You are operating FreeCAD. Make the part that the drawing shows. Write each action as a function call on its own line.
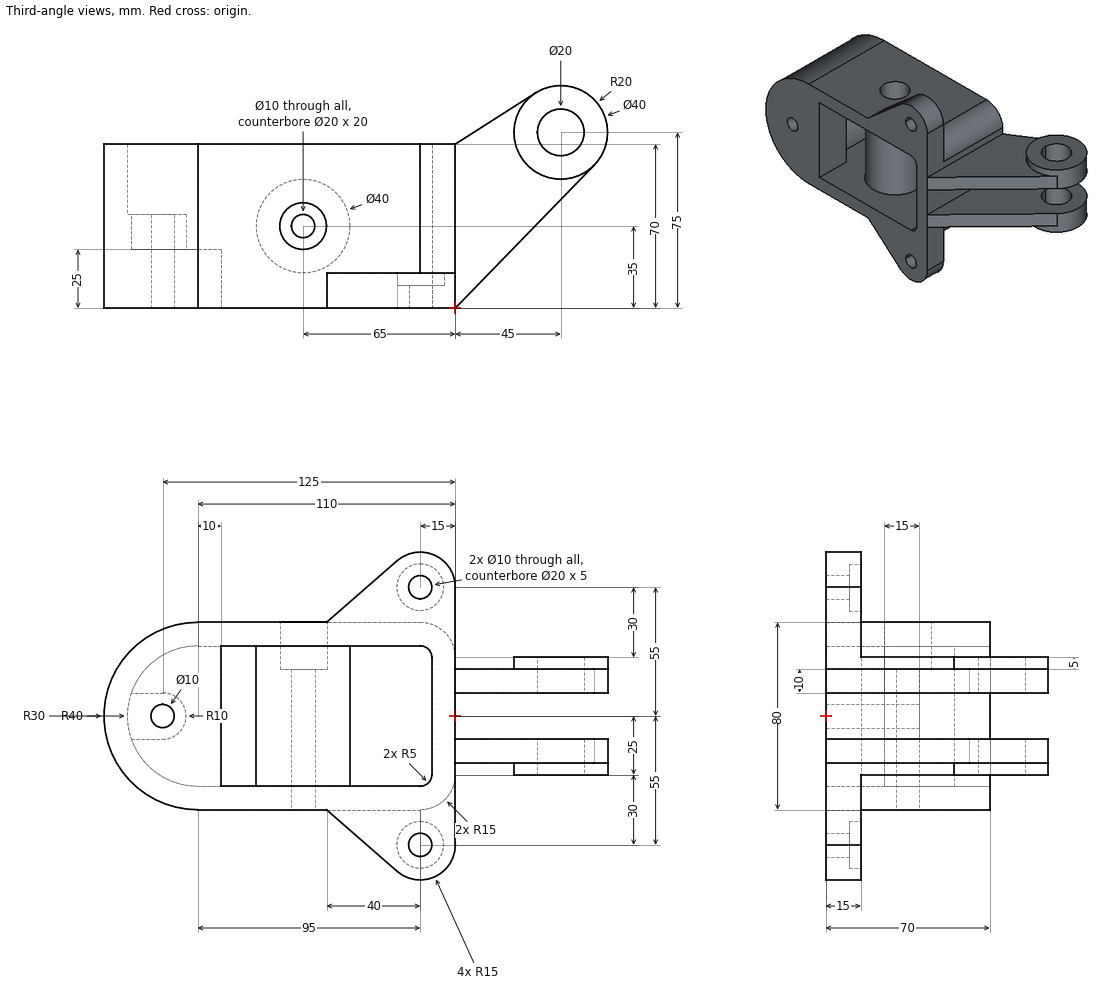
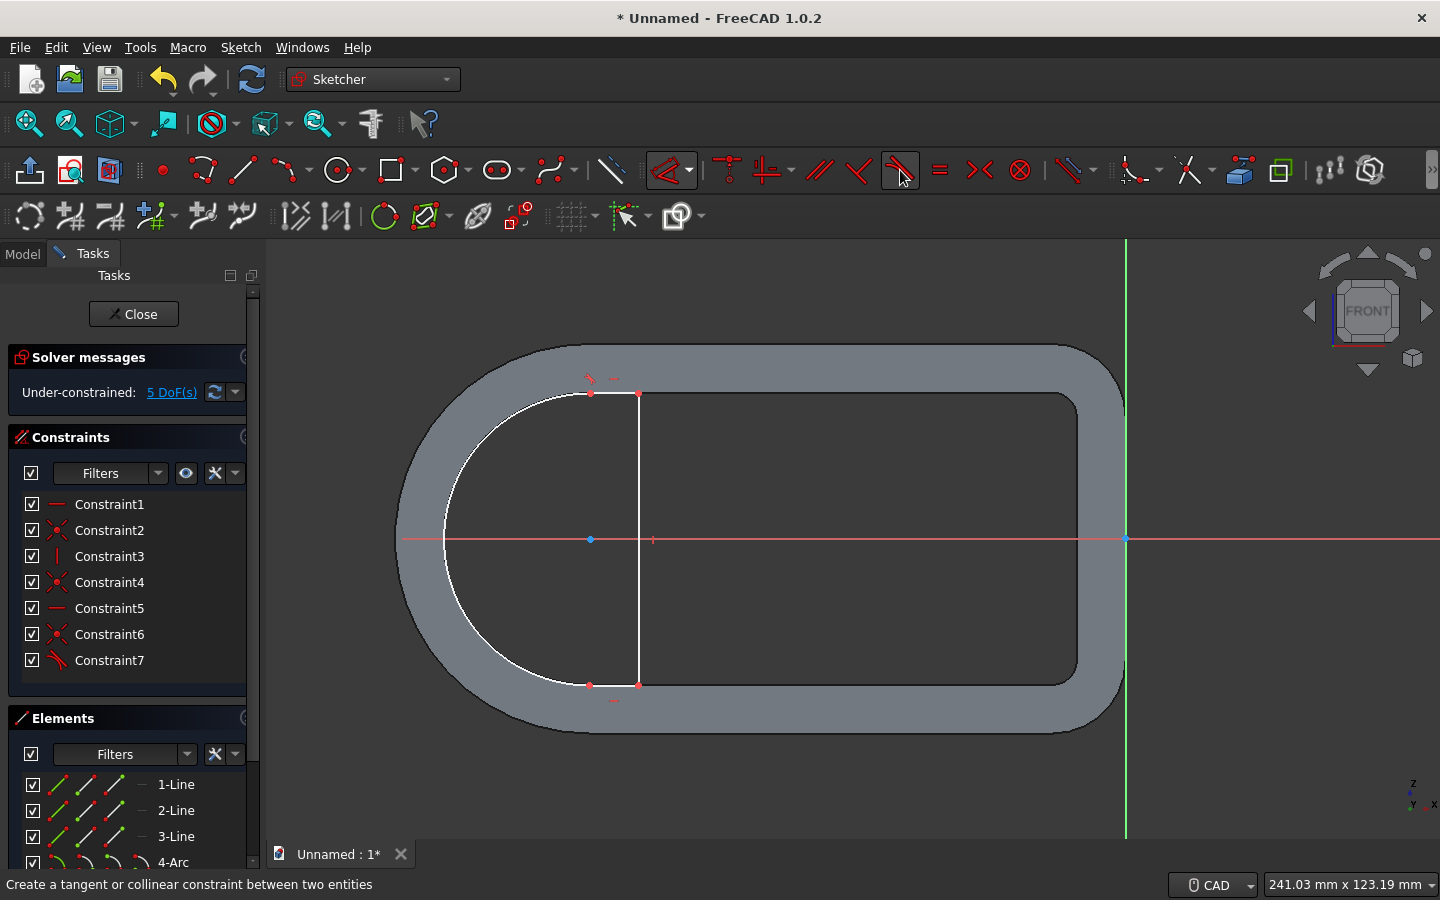
click(624, 686)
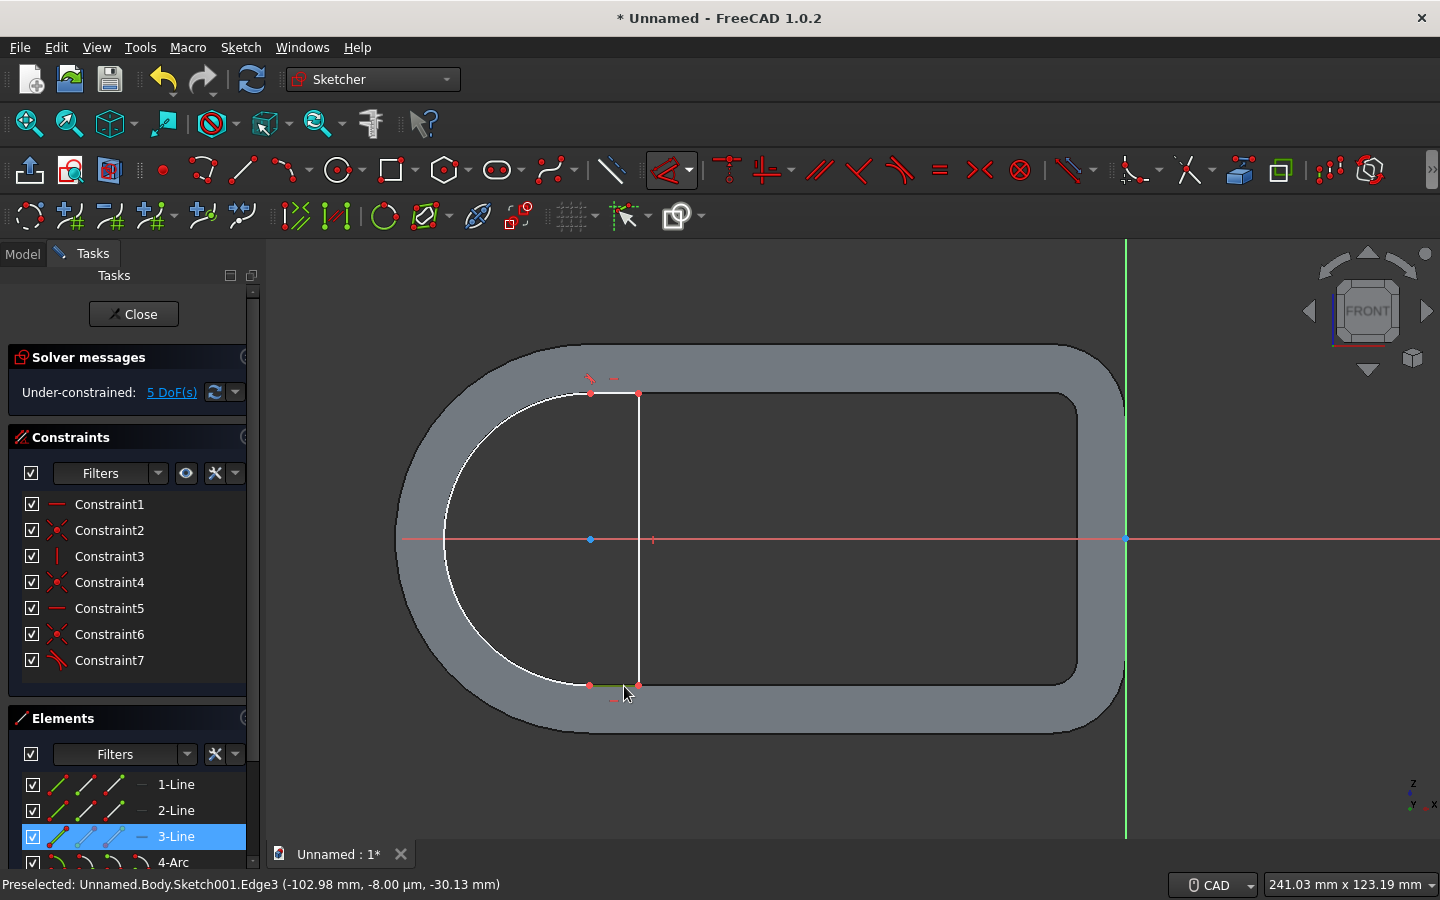
click(472, 454)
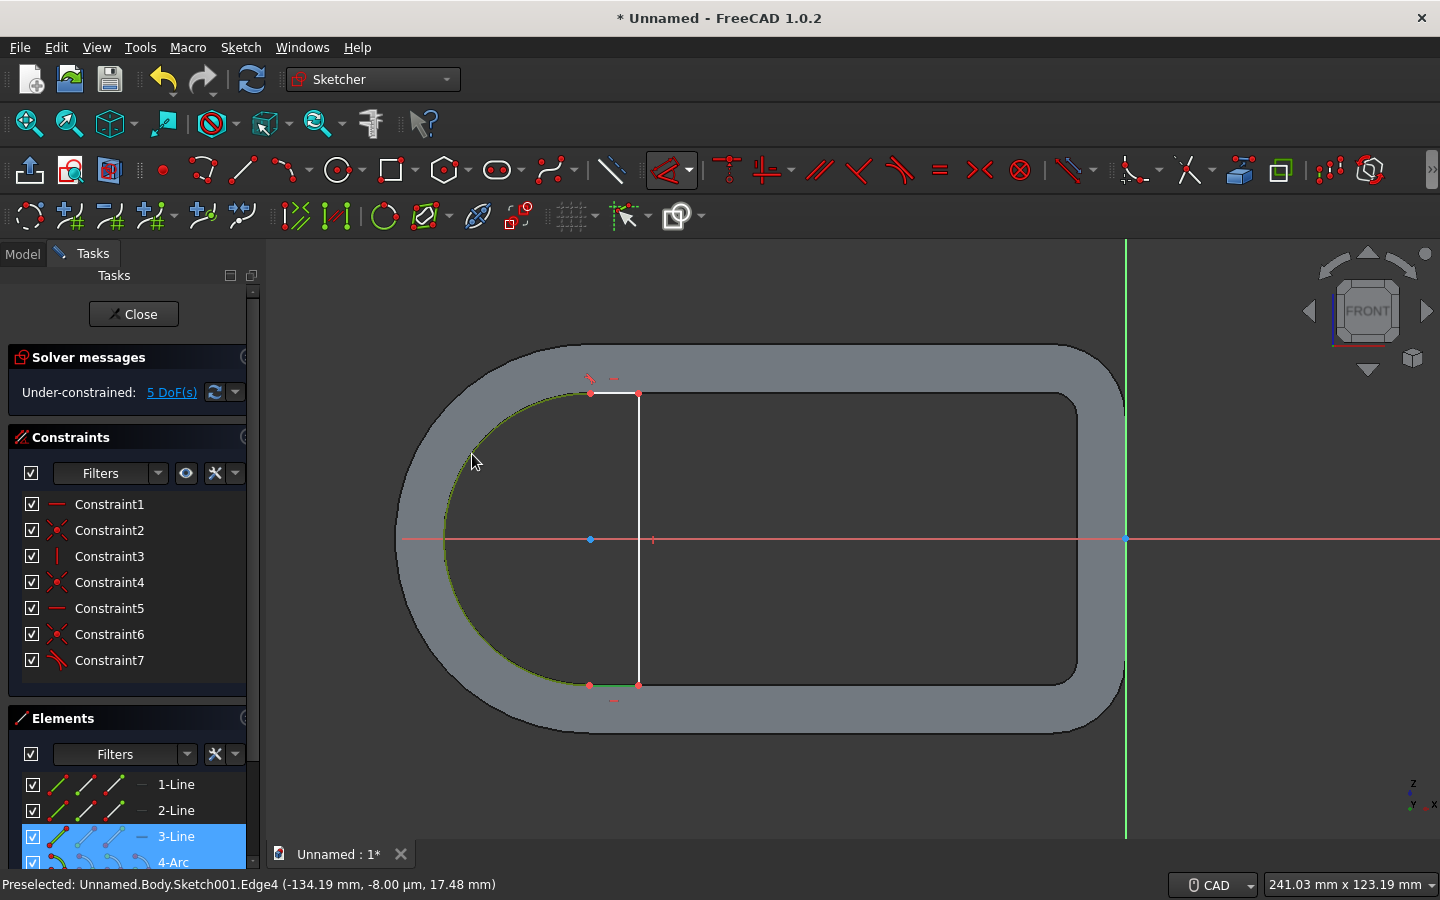
key(t)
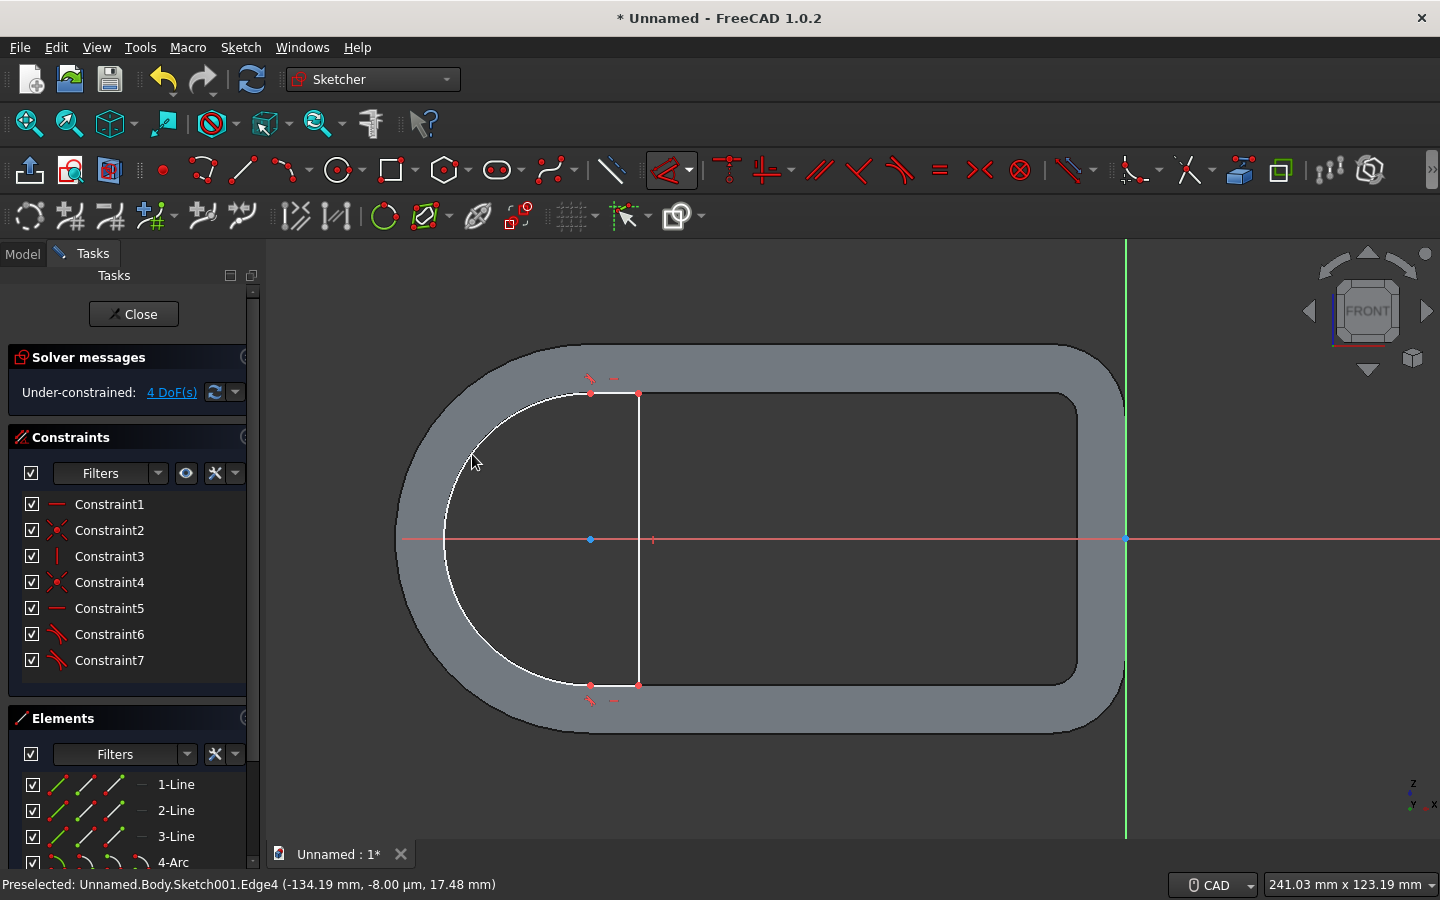
click(590, 539)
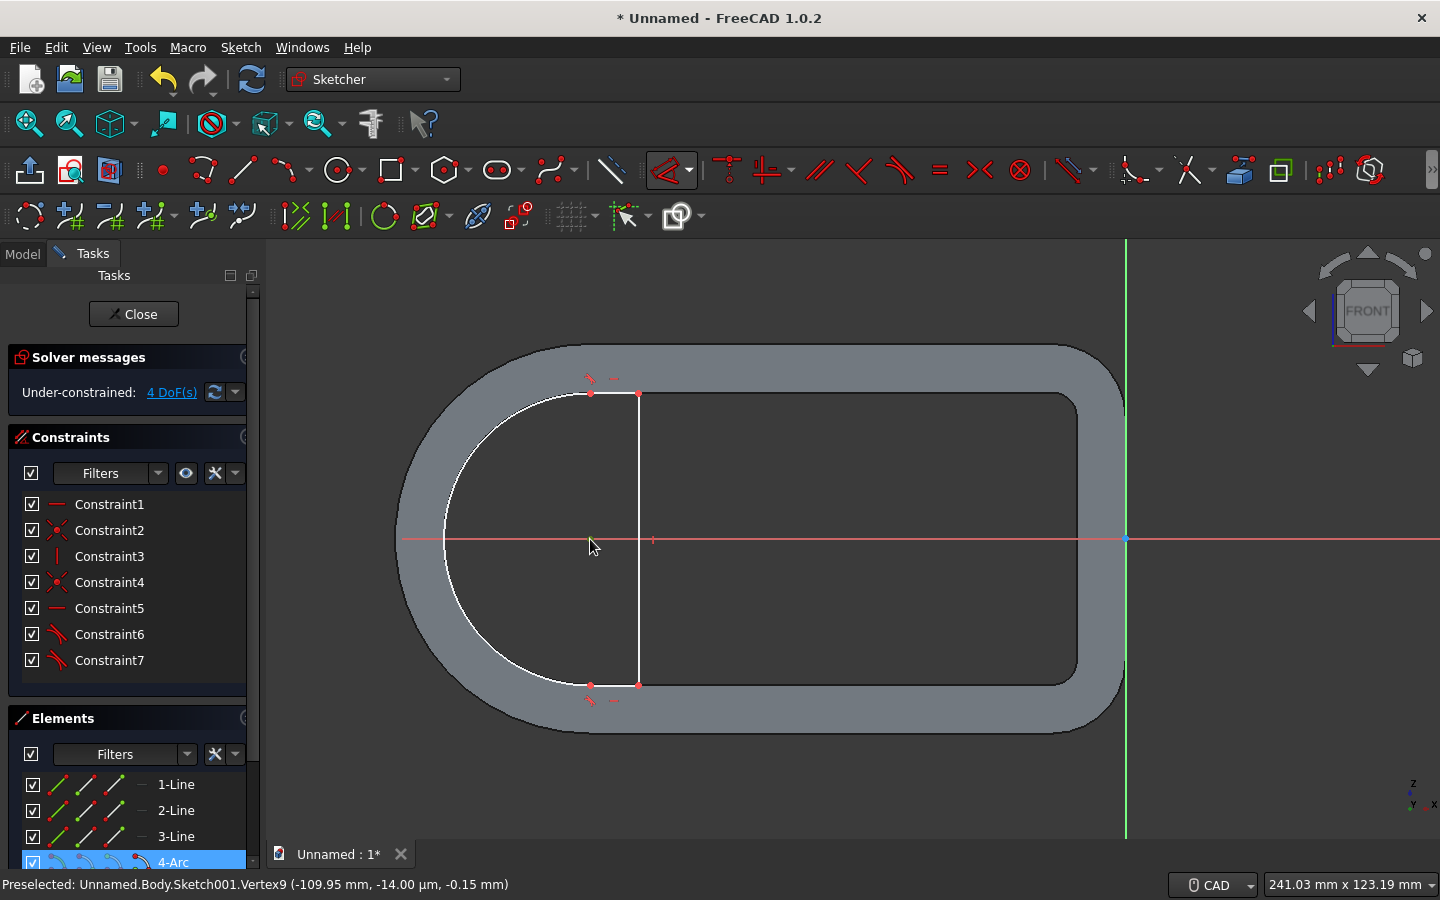
click(504, 539)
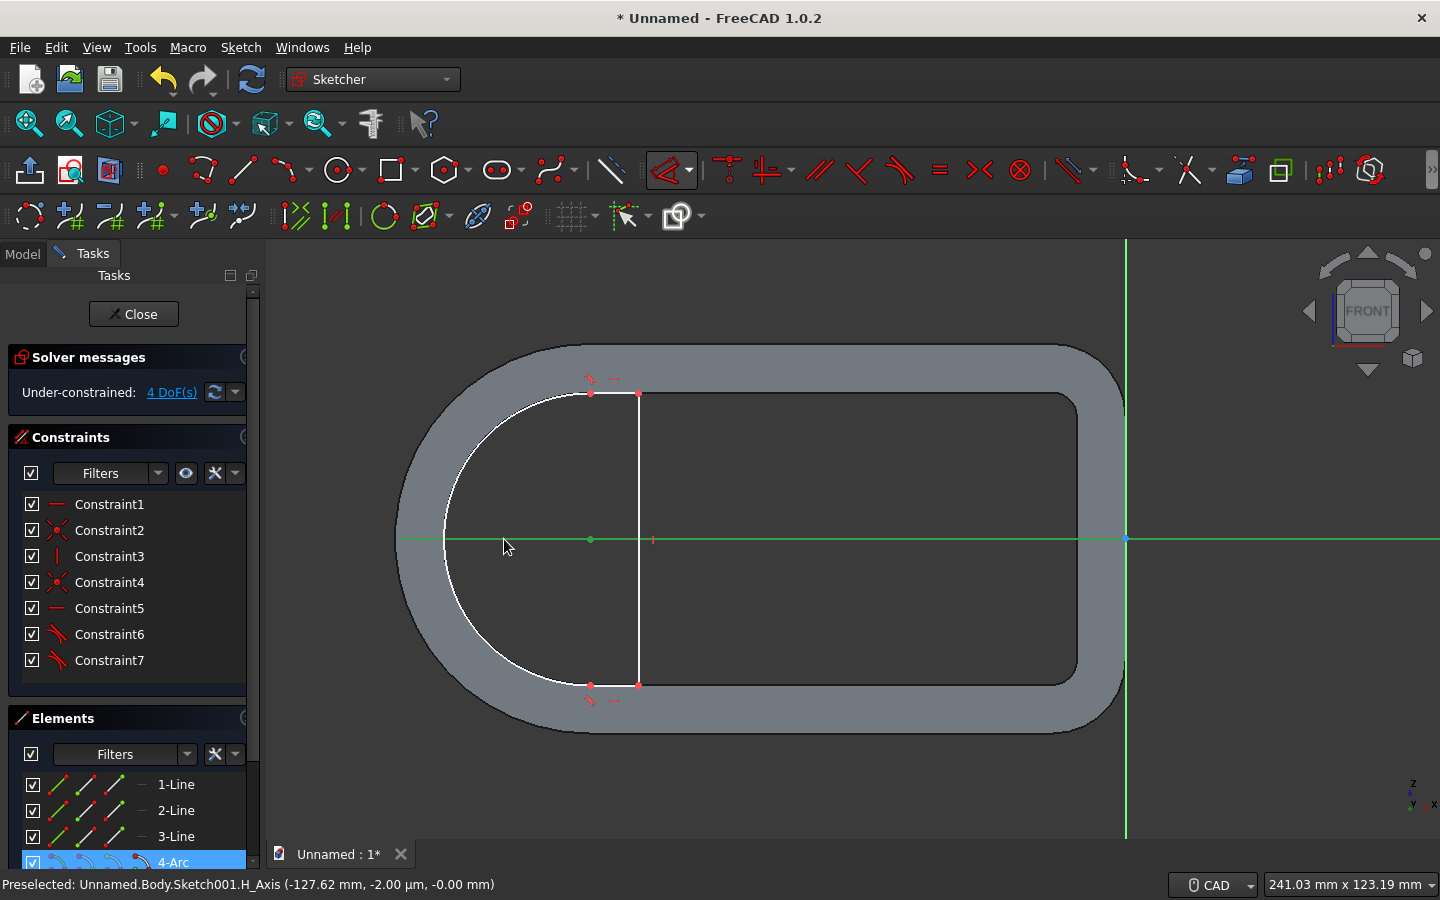
key(c)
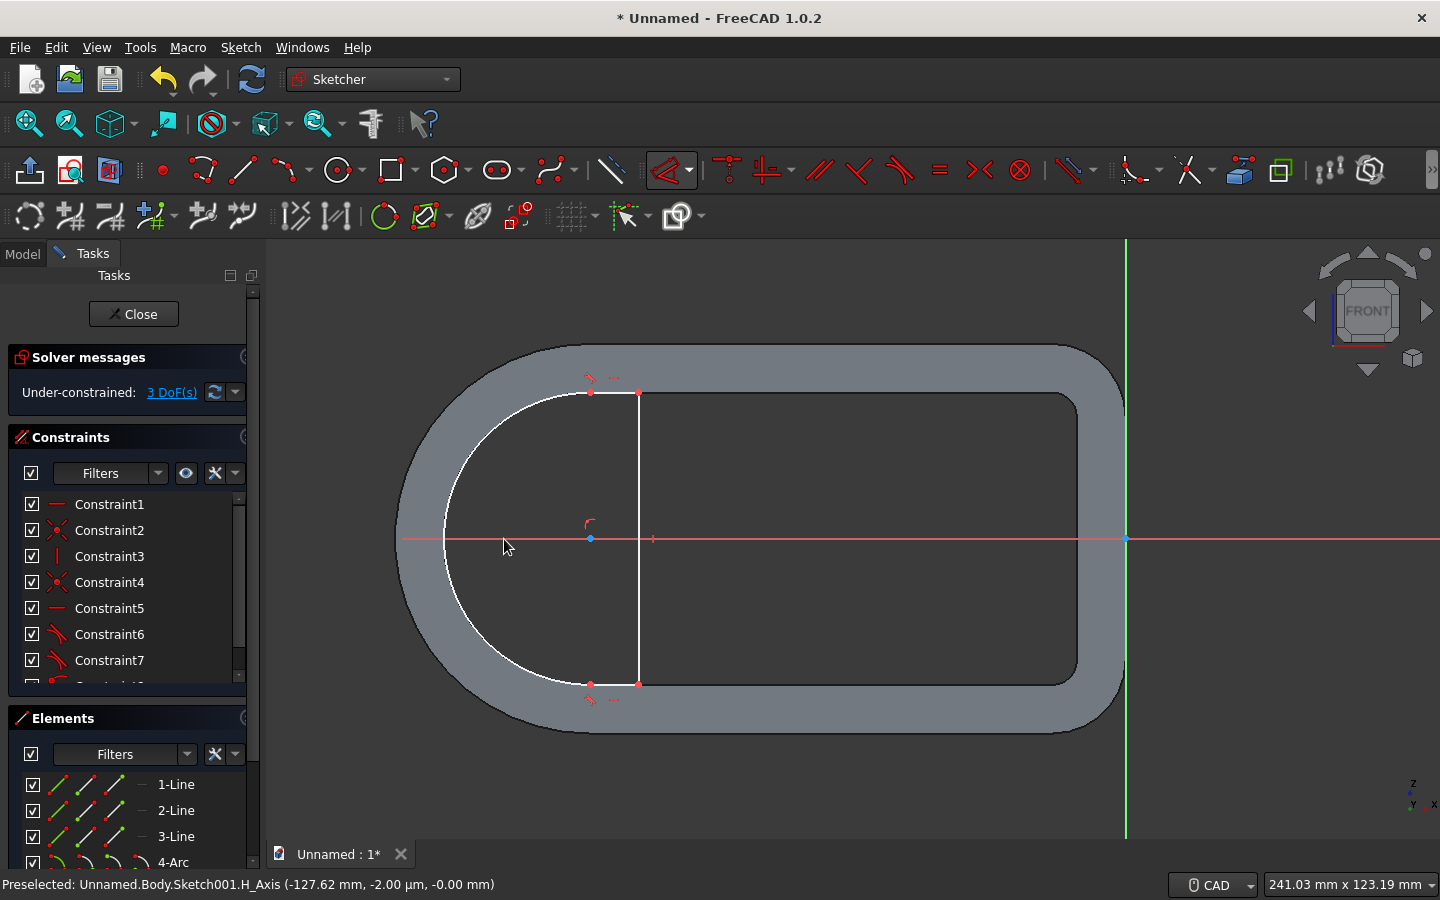
click(472, 453)